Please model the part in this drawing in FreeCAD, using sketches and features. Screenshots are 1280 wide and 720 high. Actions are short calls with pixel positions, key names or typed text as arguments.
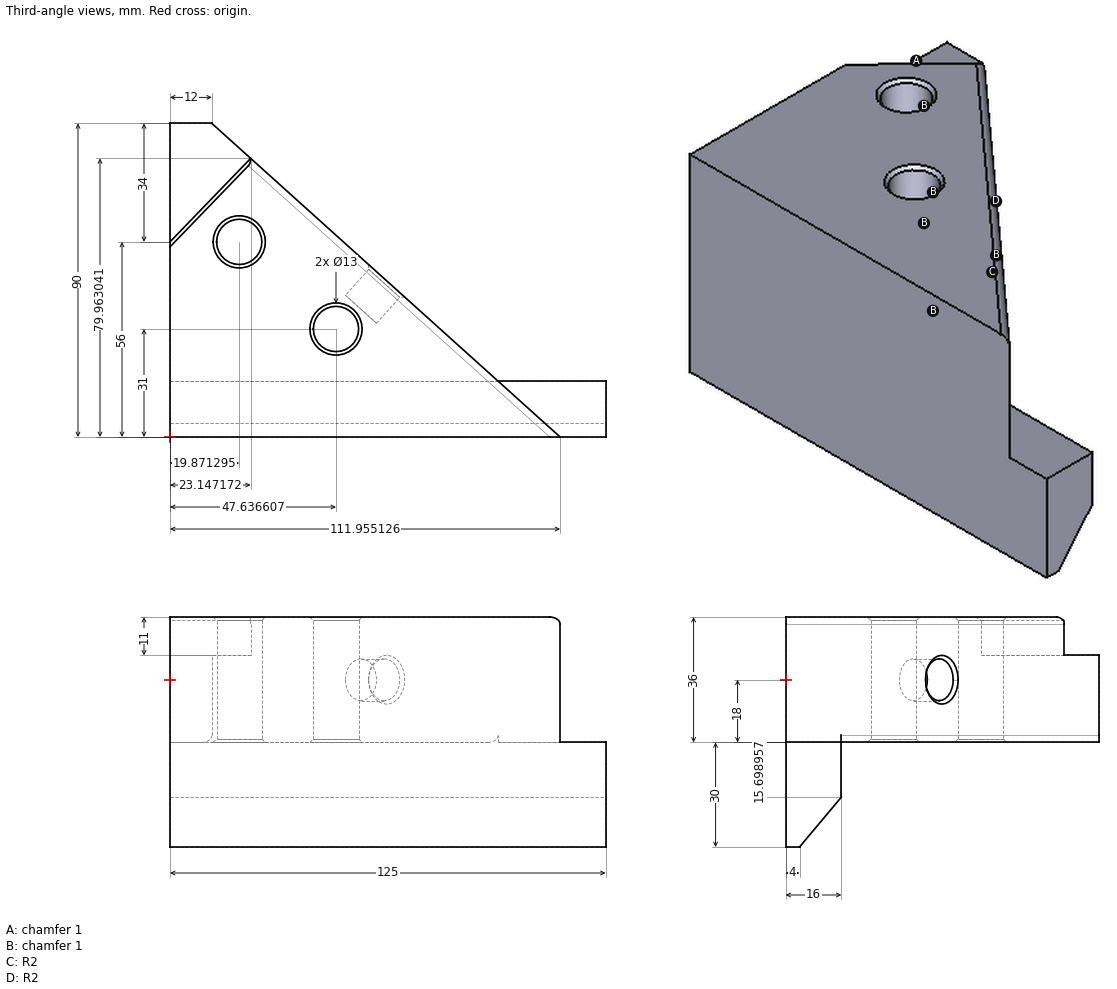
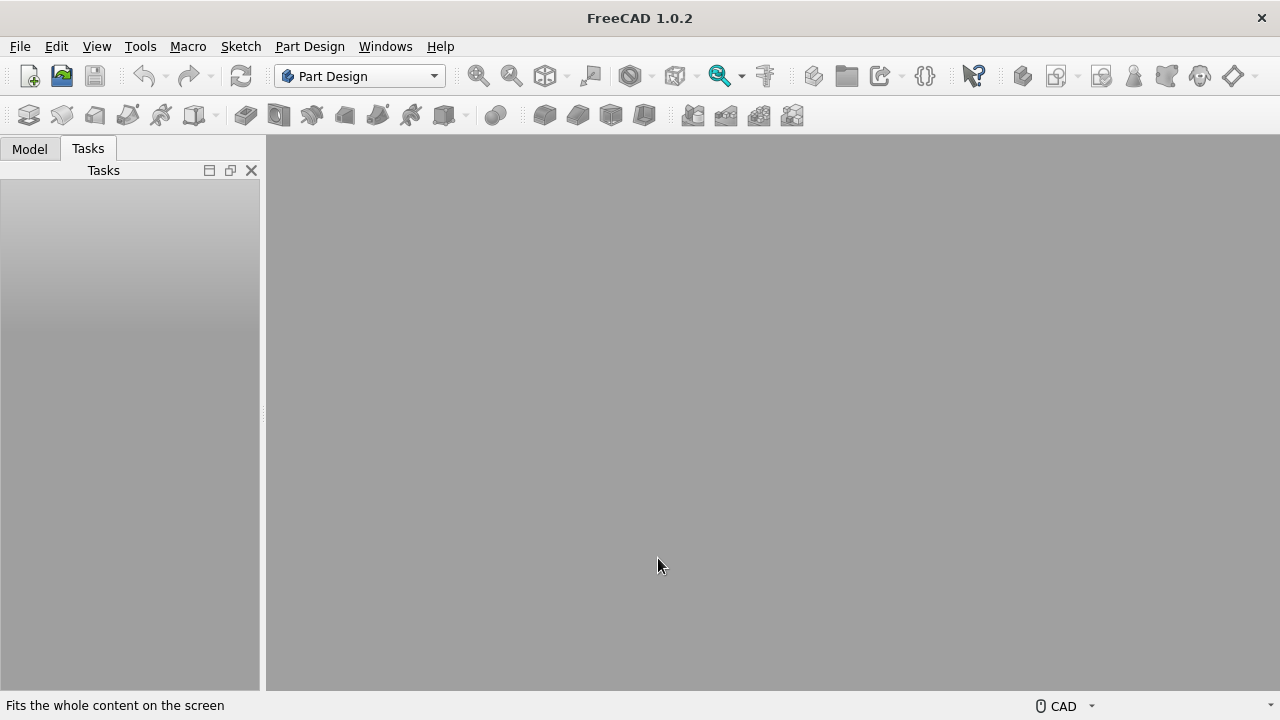
key(ctrl+n)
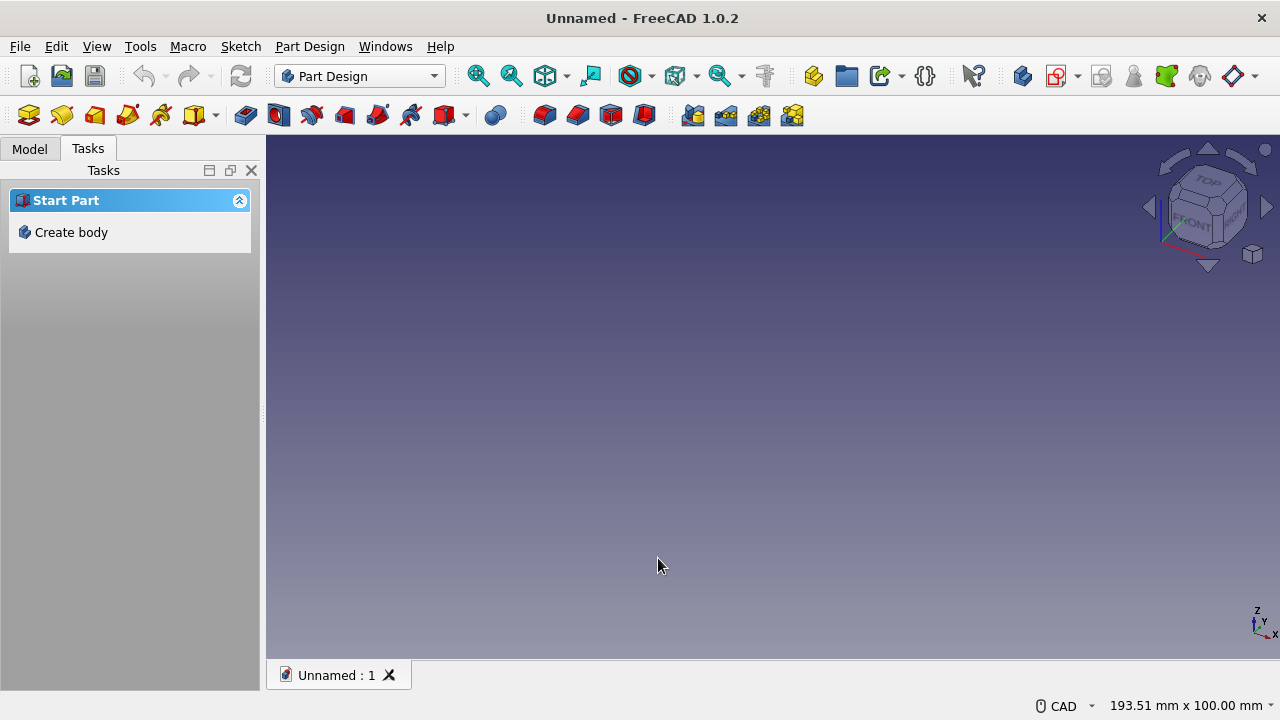
click(1056, 76)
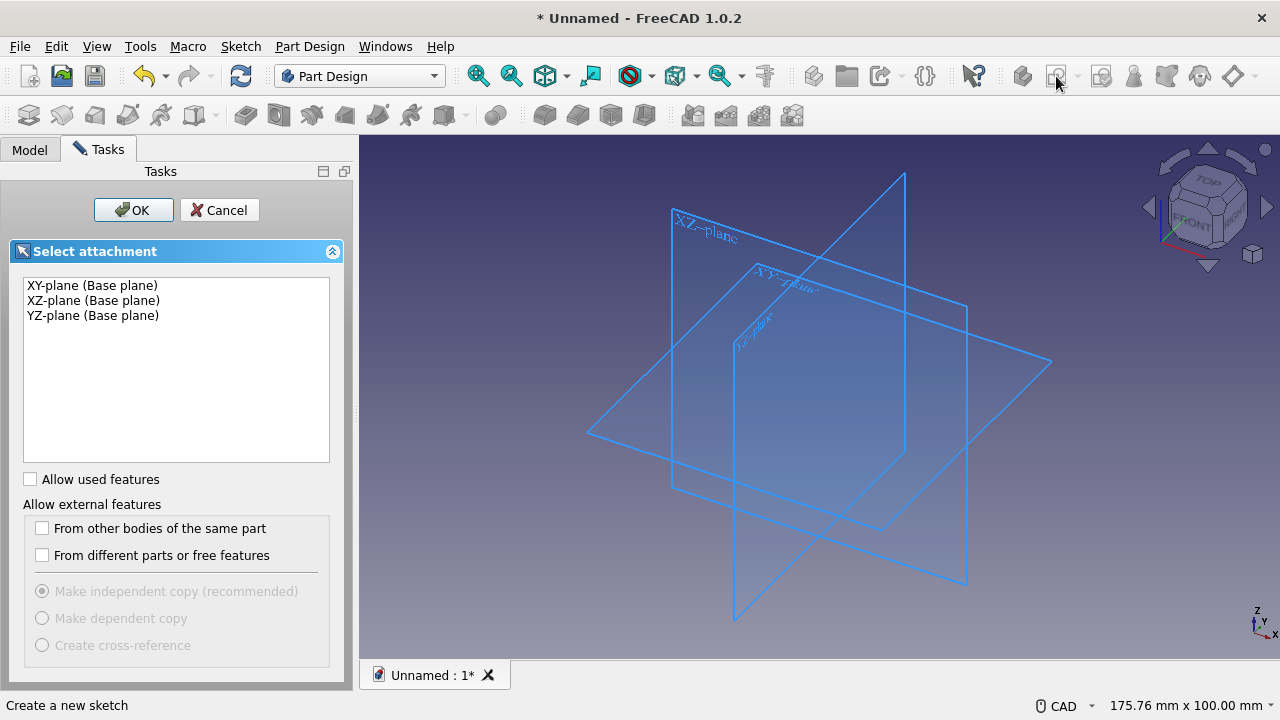
click(84, 286)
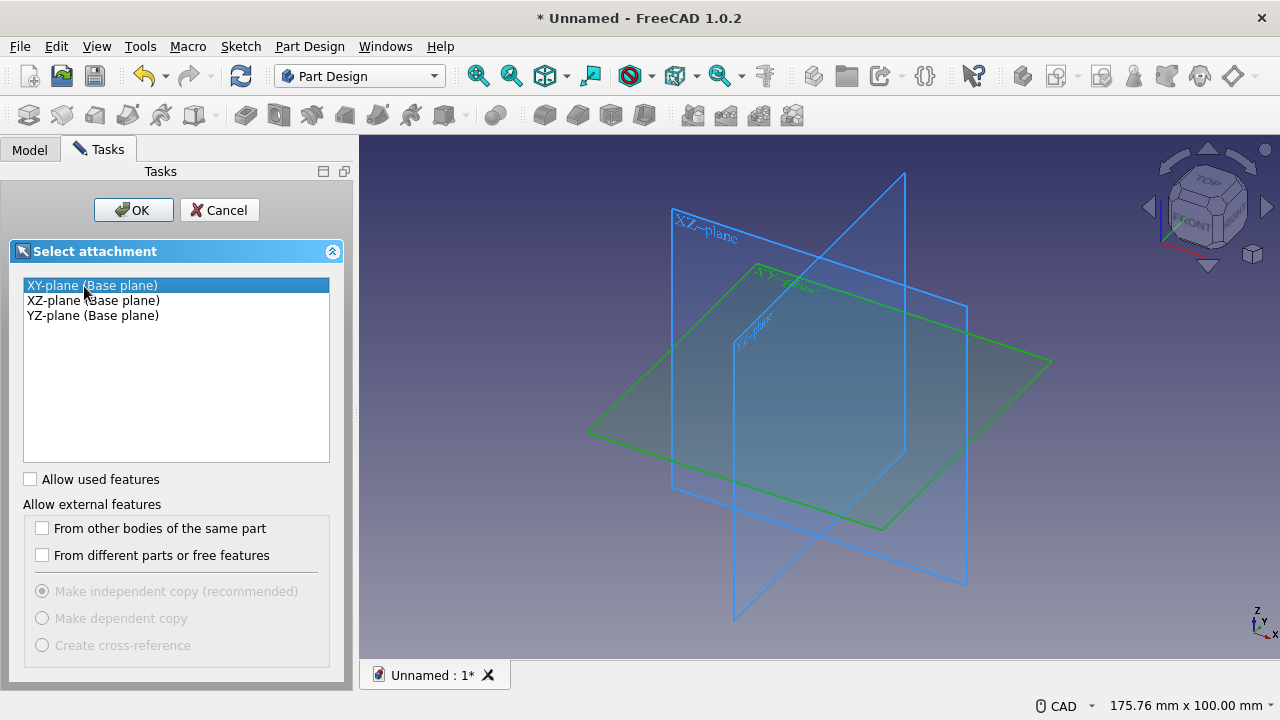
click(134, 210)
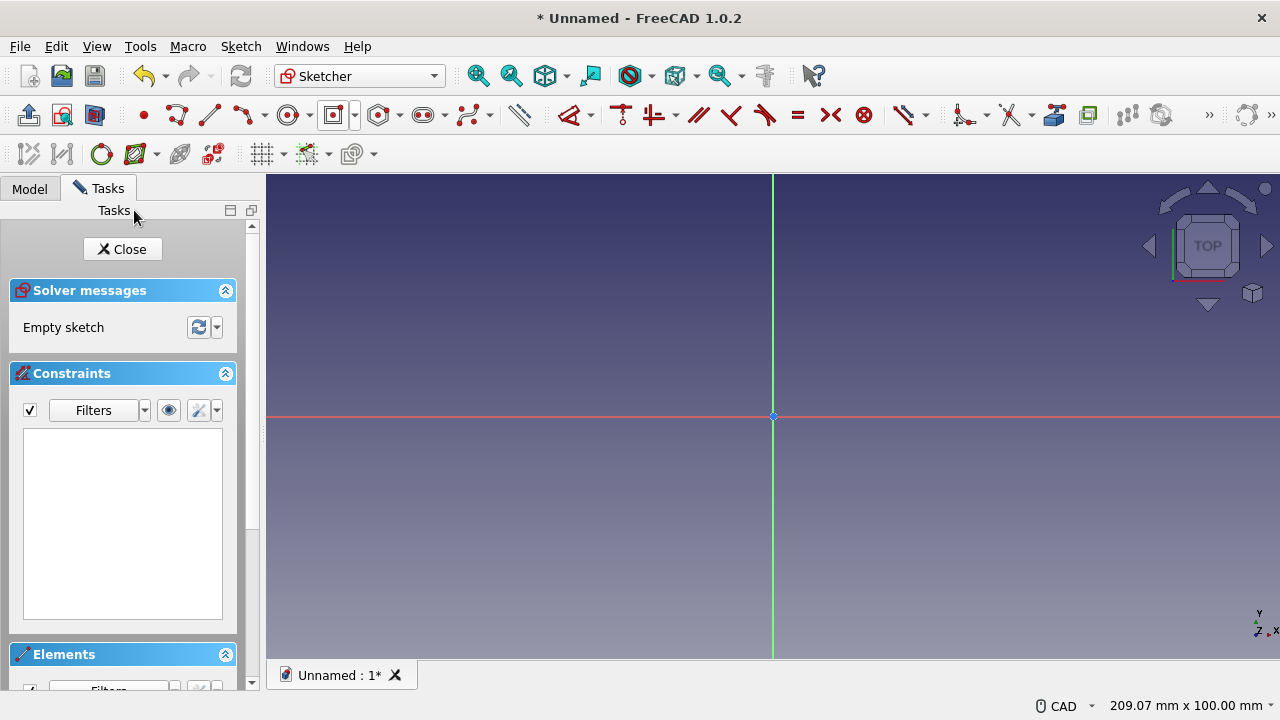
scroll(294, 631, down, 3)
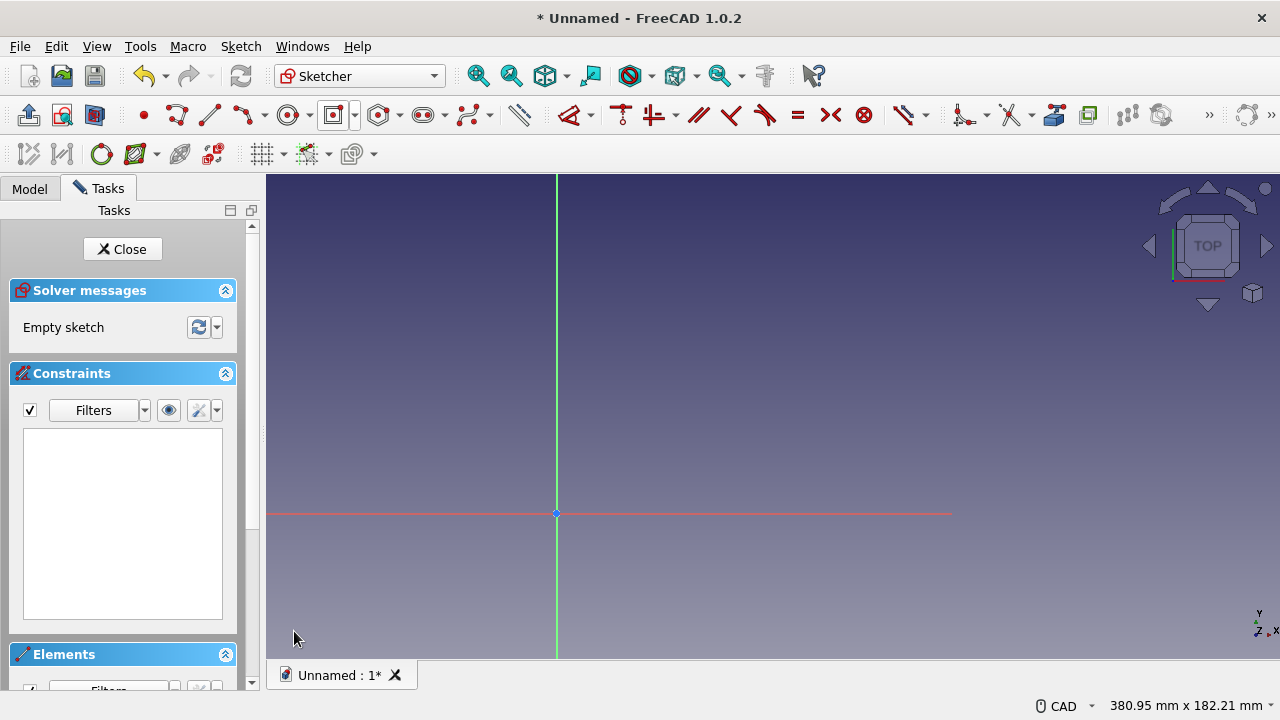
click(177, 116)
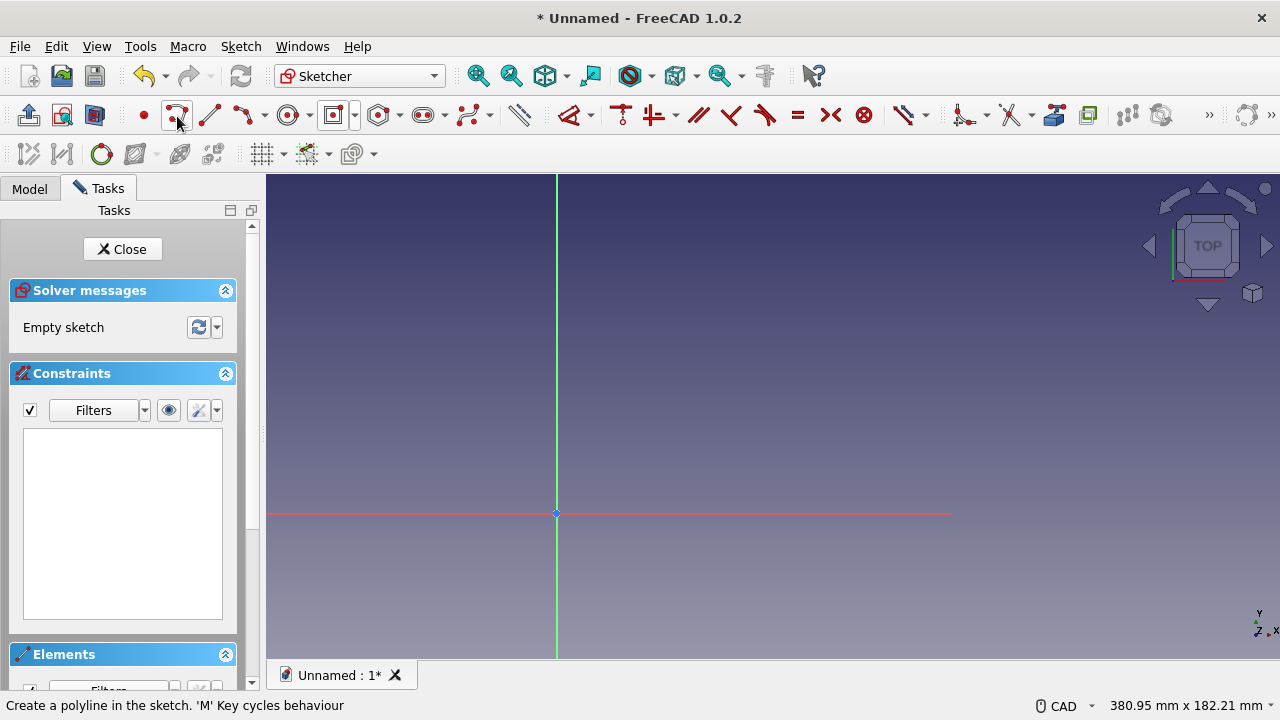
click(557, 514)
click(855, 505)
click(589, 274)
click(566, 274)
click(557, 514)
key(Escape)
key(Escape)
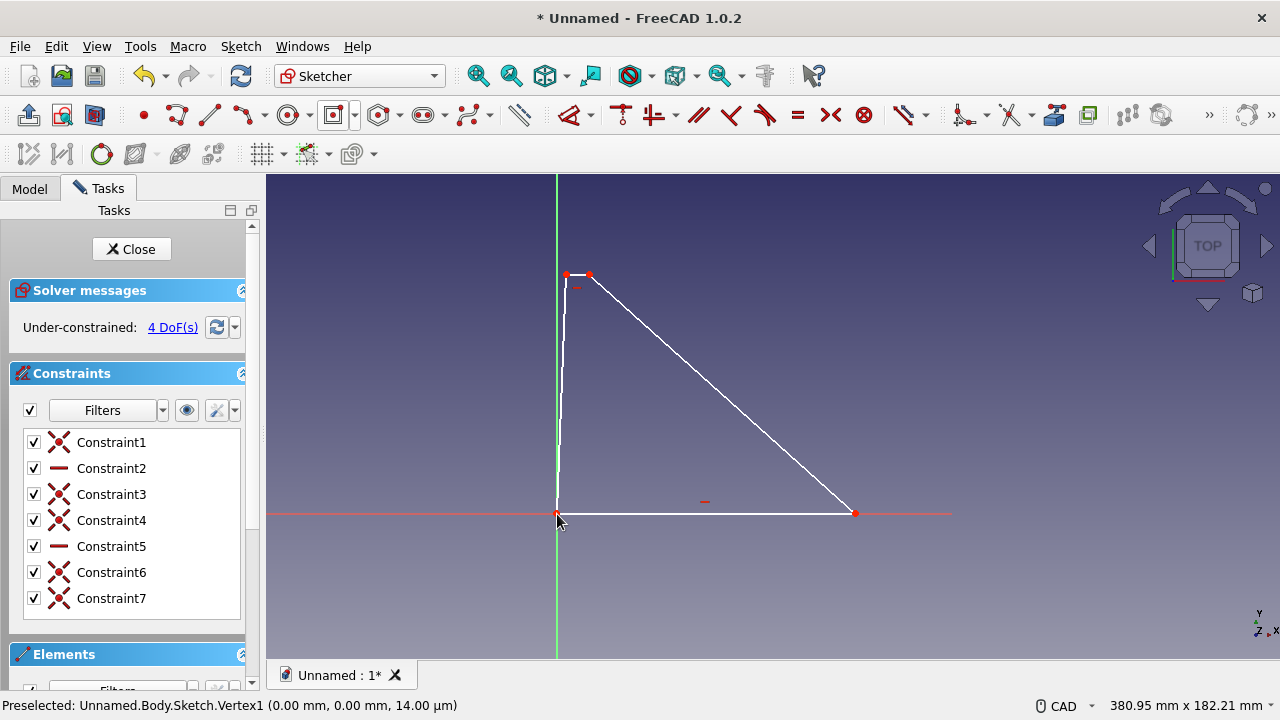
click(560, 442)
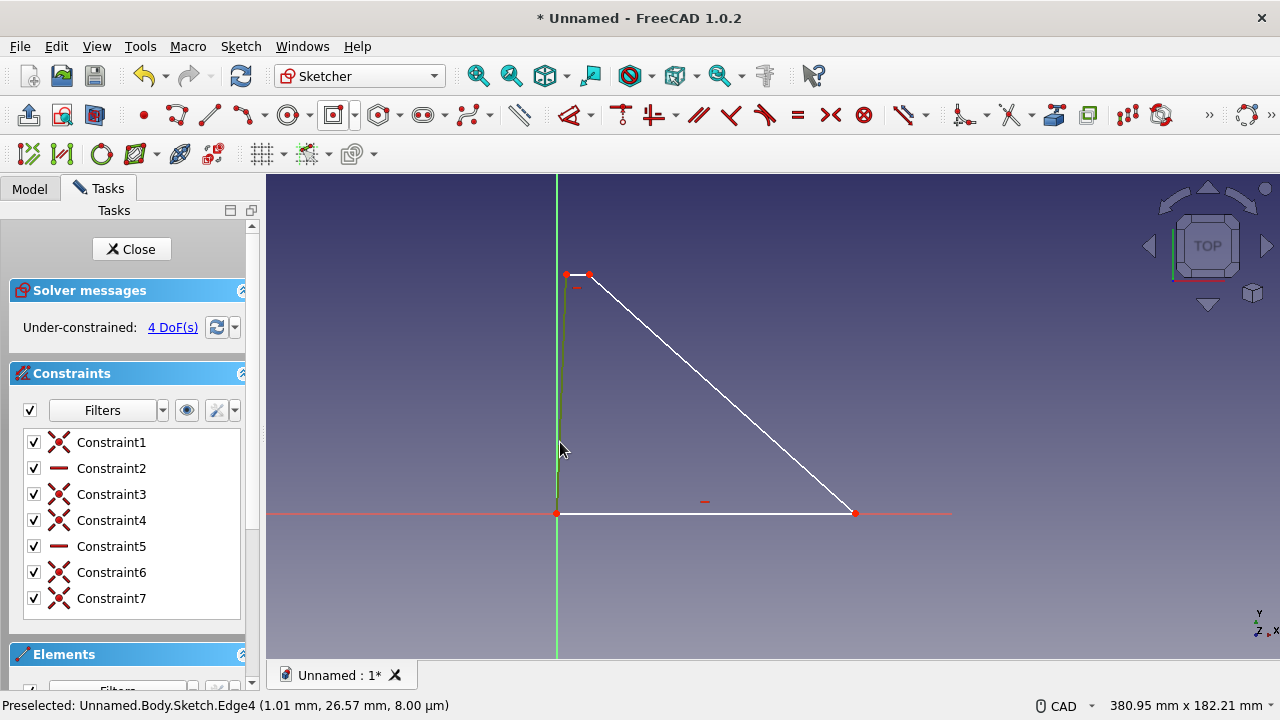
key(v)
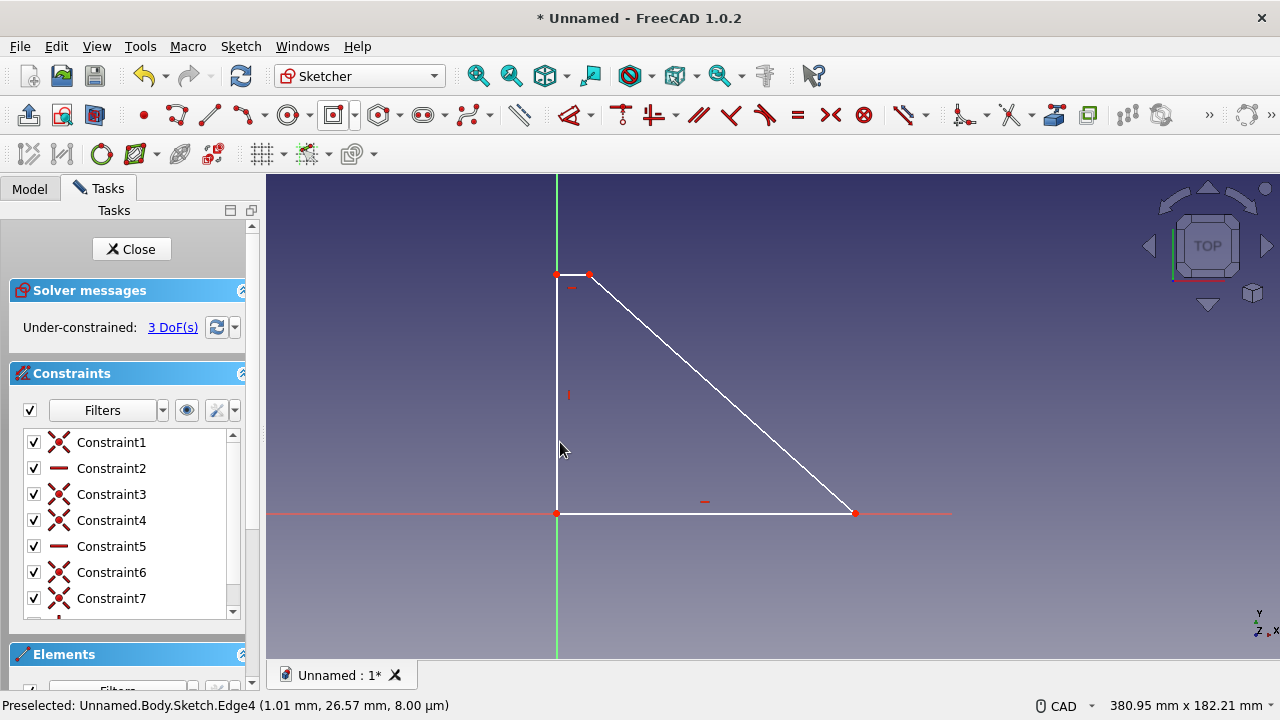
click(568, 116)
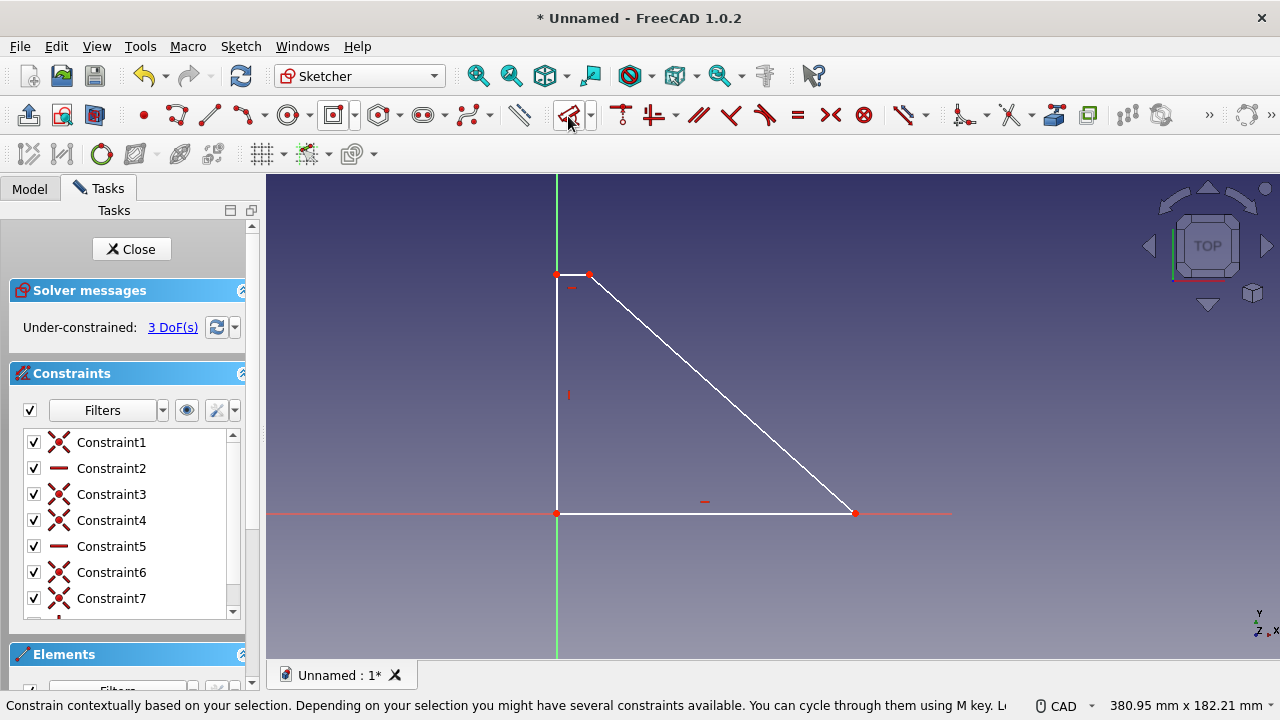
scroll(579, 275, up, 2)